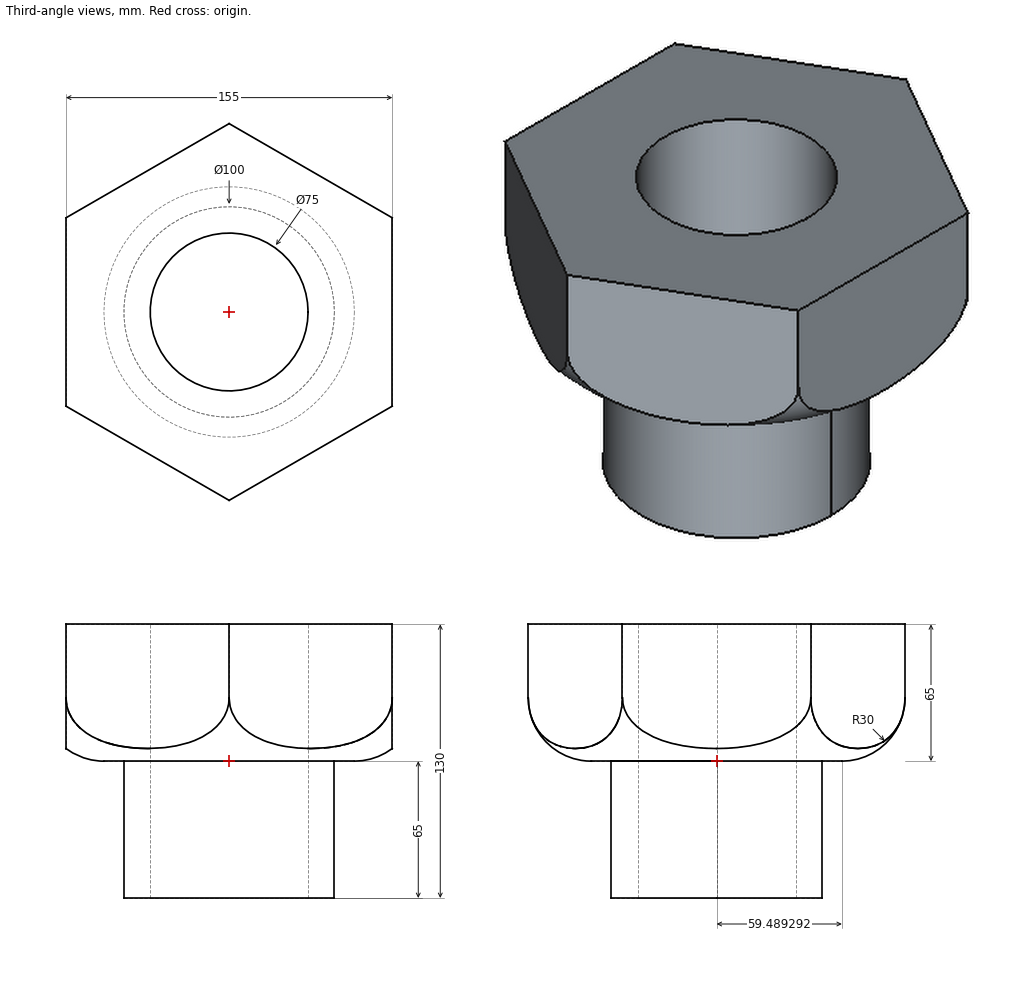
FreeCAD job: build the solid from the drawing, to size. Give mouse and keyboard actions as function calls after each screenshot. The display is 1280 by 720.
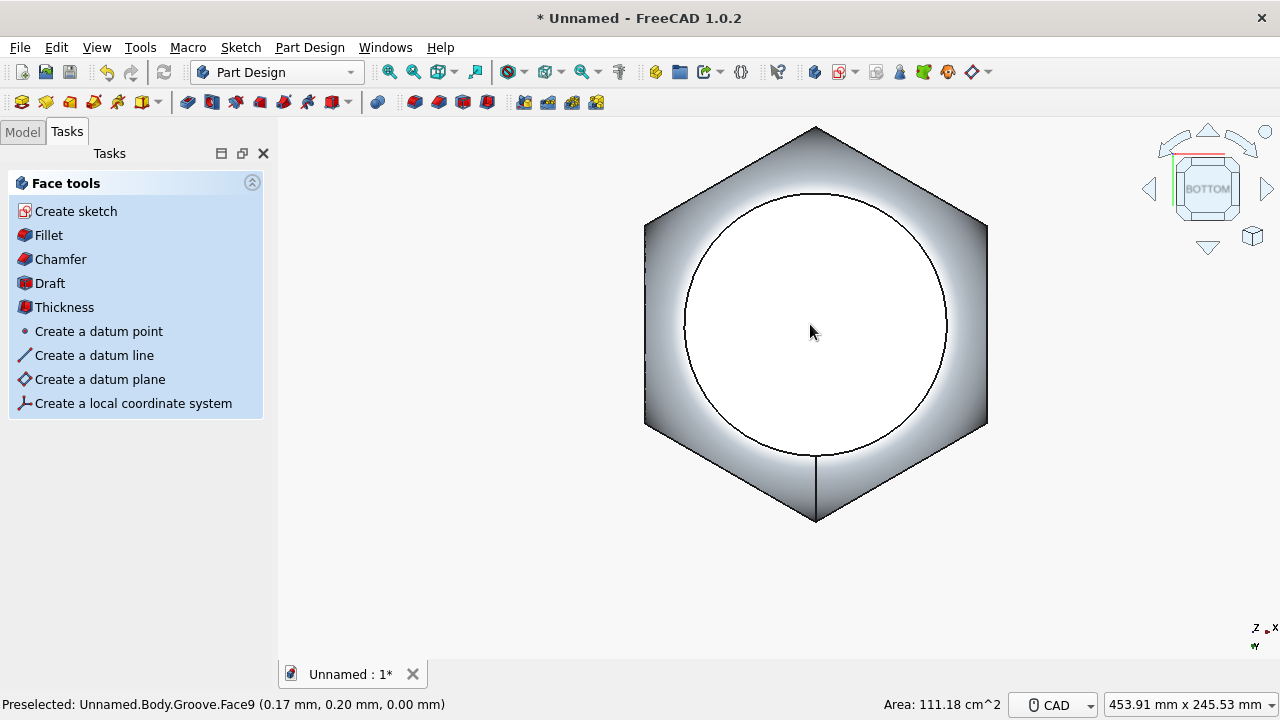
click(840, 72)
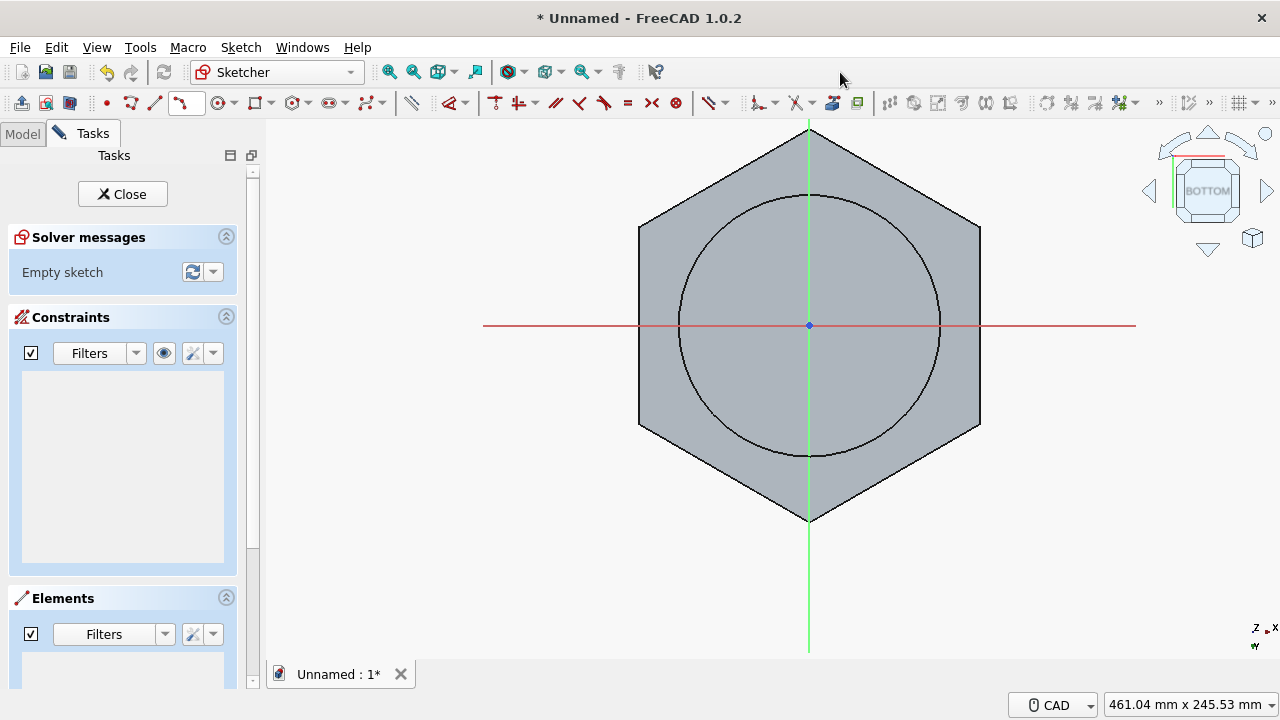
scroll(1023, 197, up, 2)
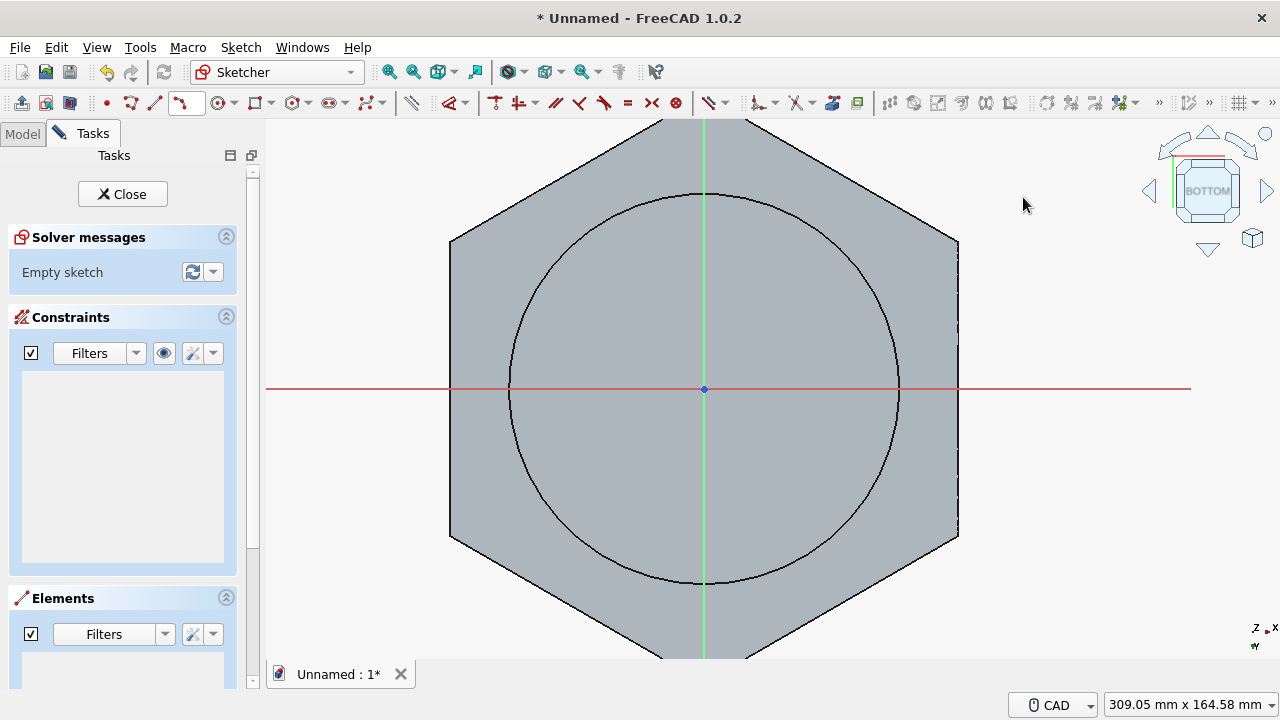
key(g)
key(c)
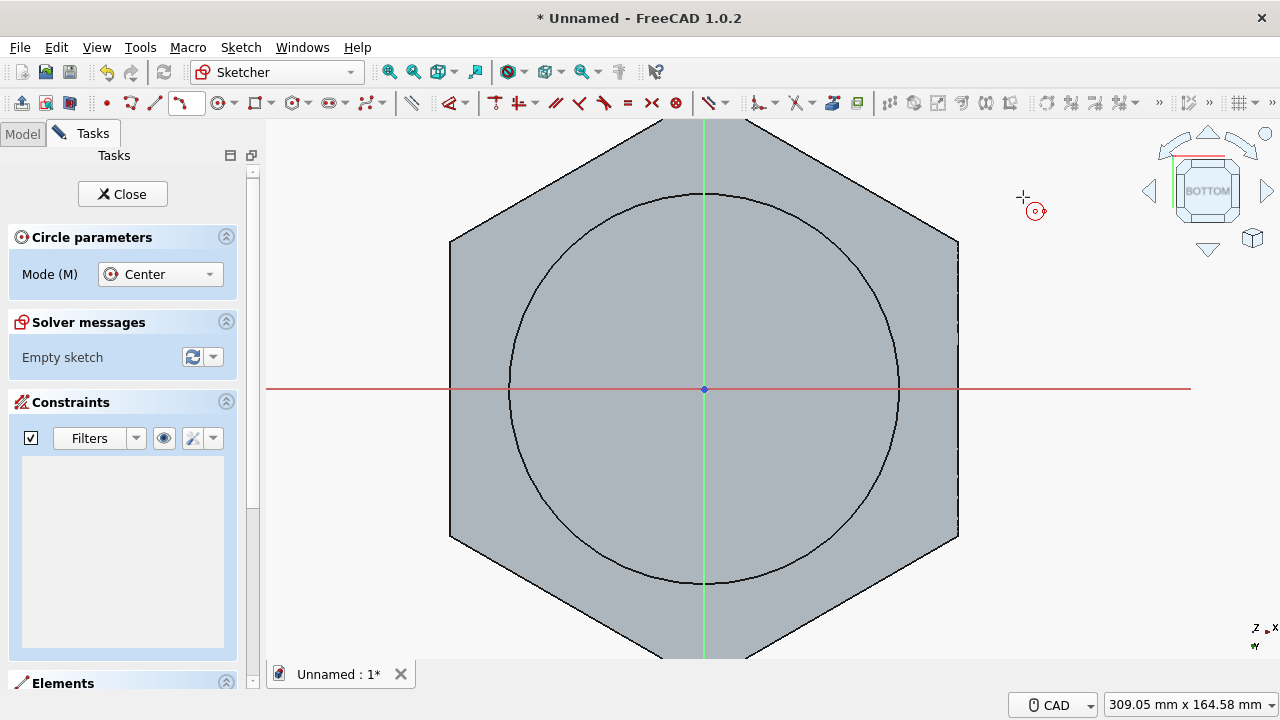
click(704, 389)
move(820, 273)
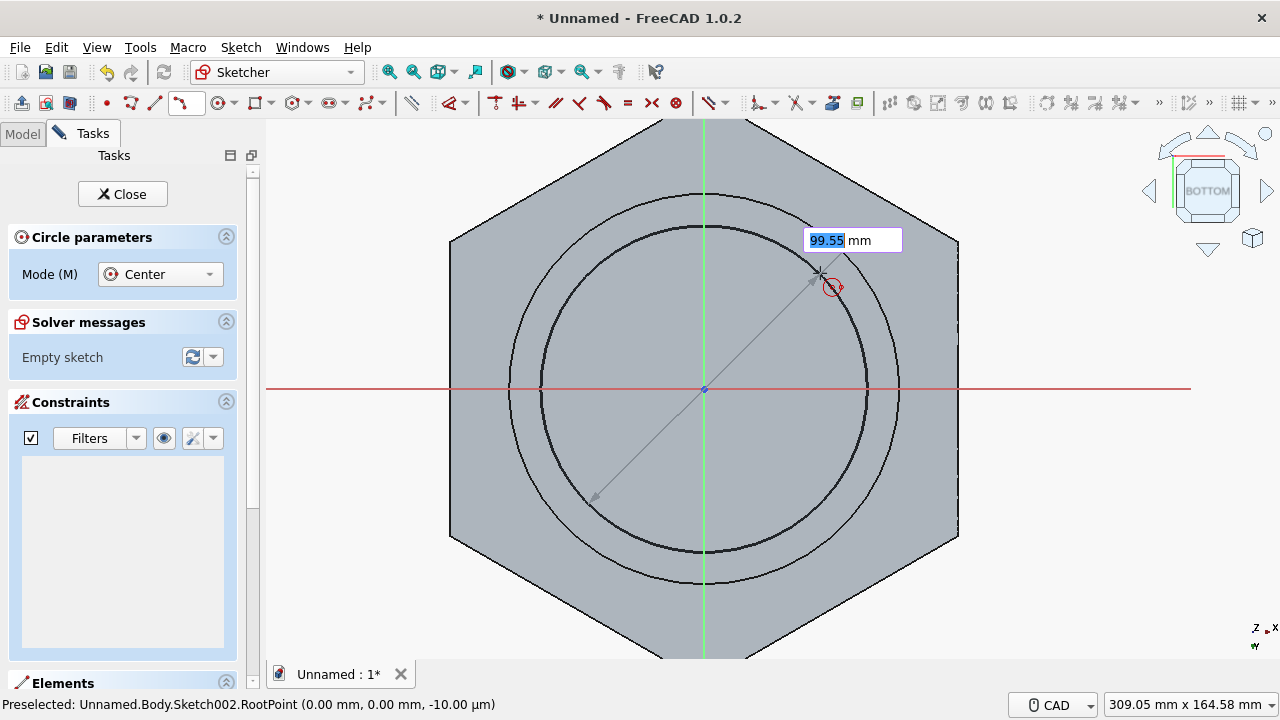
text(100)
key(Return)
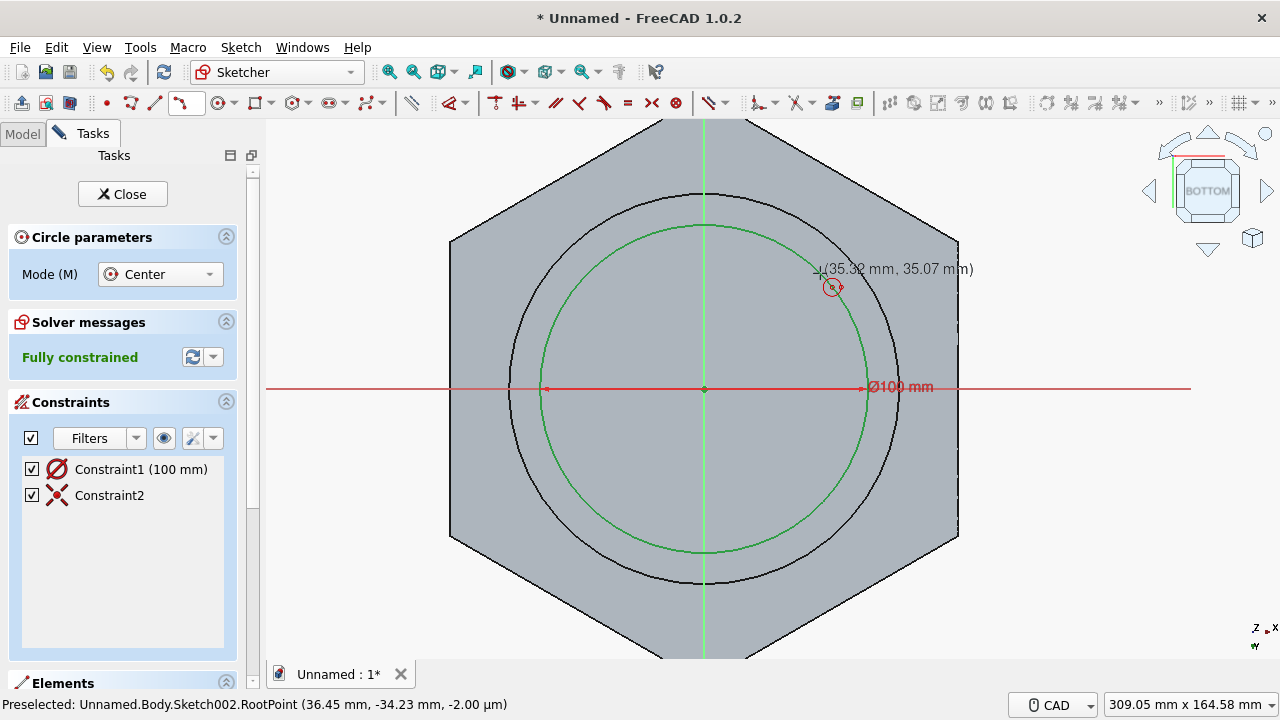
click(704, 389)
move(791, 302)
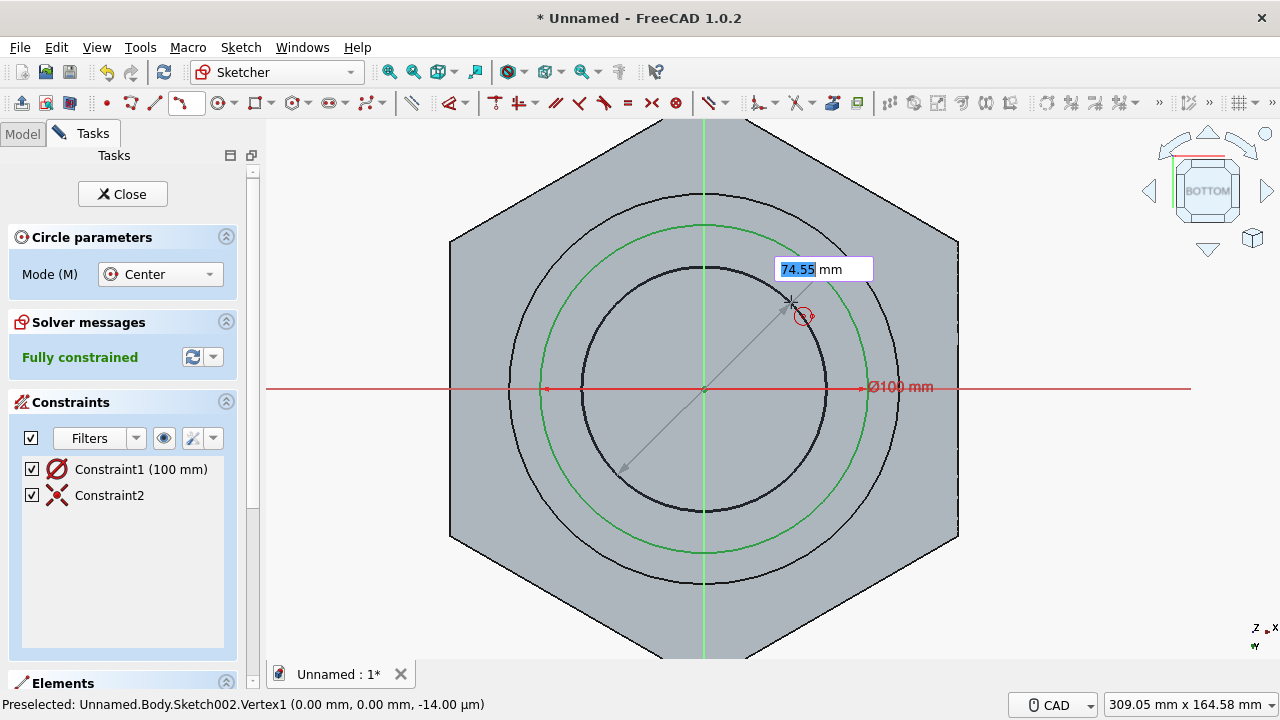
text(75)
key(Return)
key(Escape)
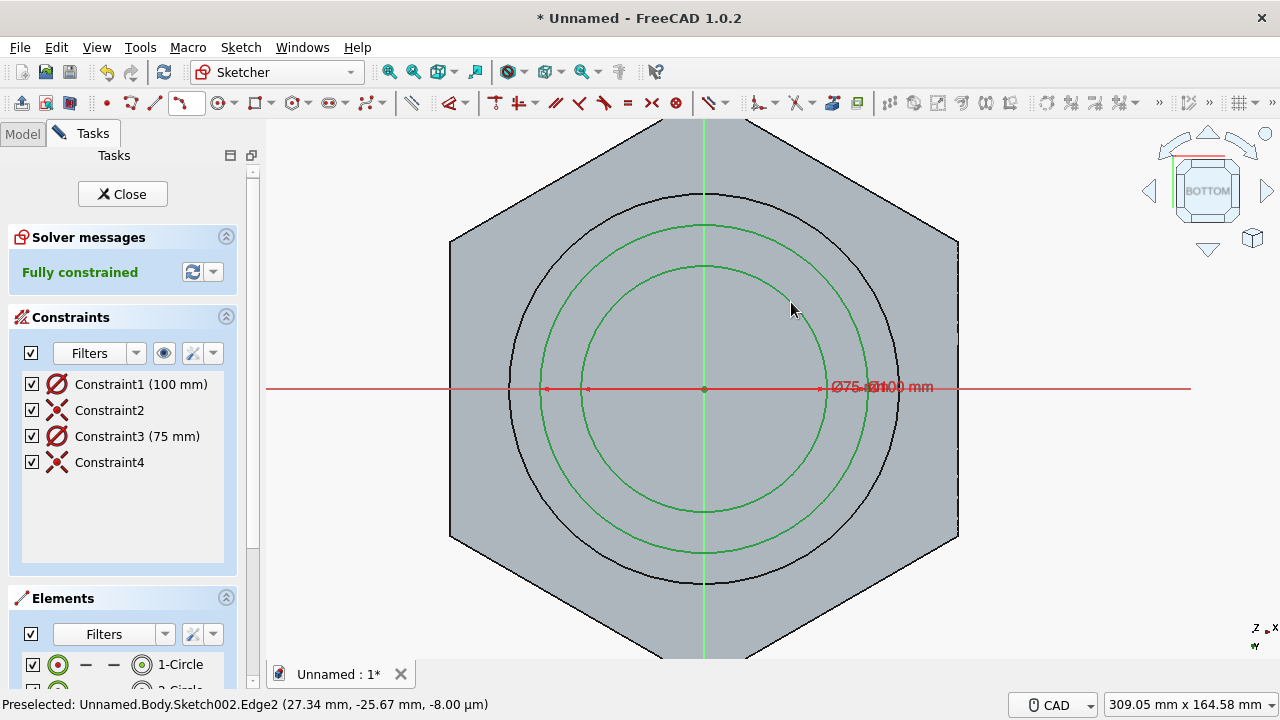
click(123, 194)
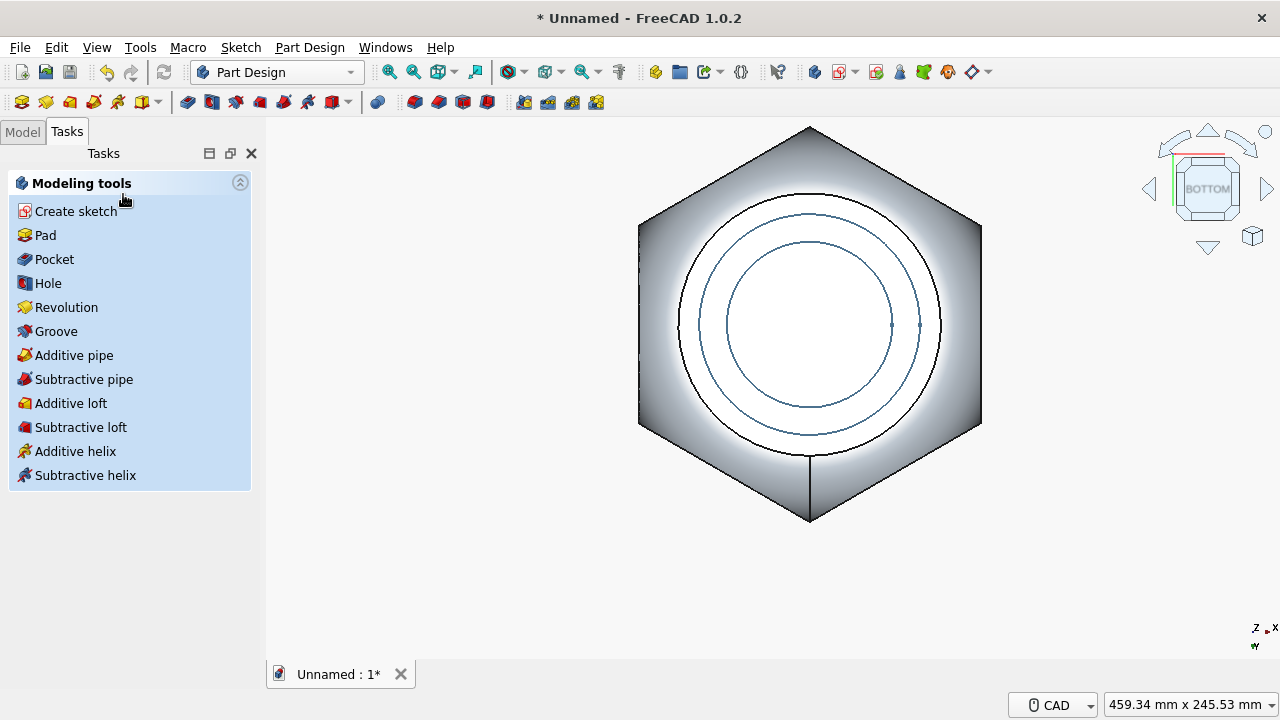
click(22, 102)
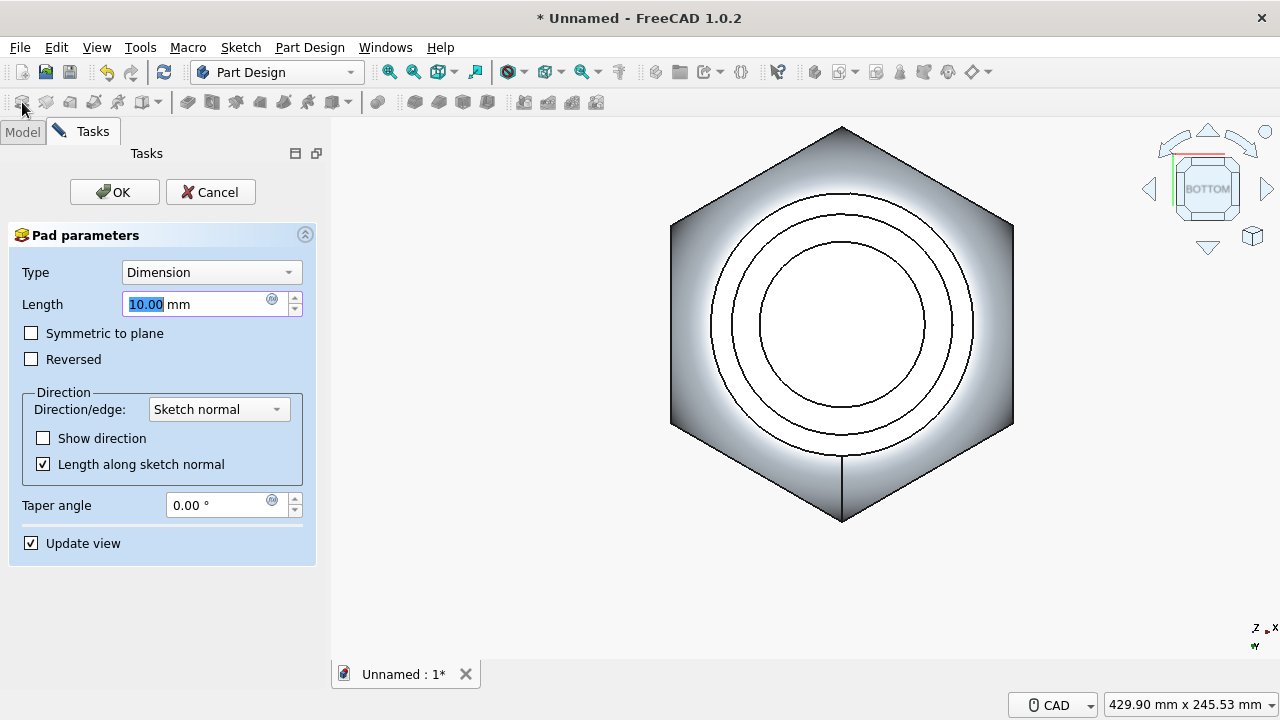
text(65)
key(Tab)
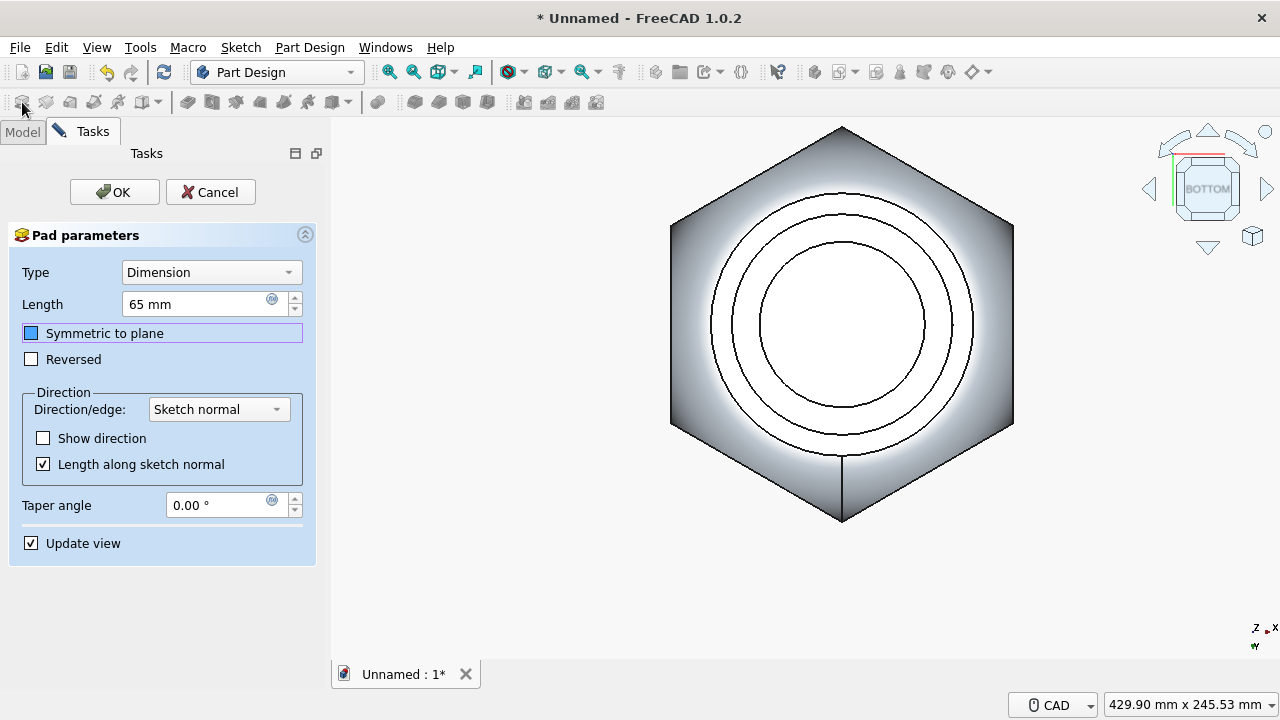
click(115, 192)